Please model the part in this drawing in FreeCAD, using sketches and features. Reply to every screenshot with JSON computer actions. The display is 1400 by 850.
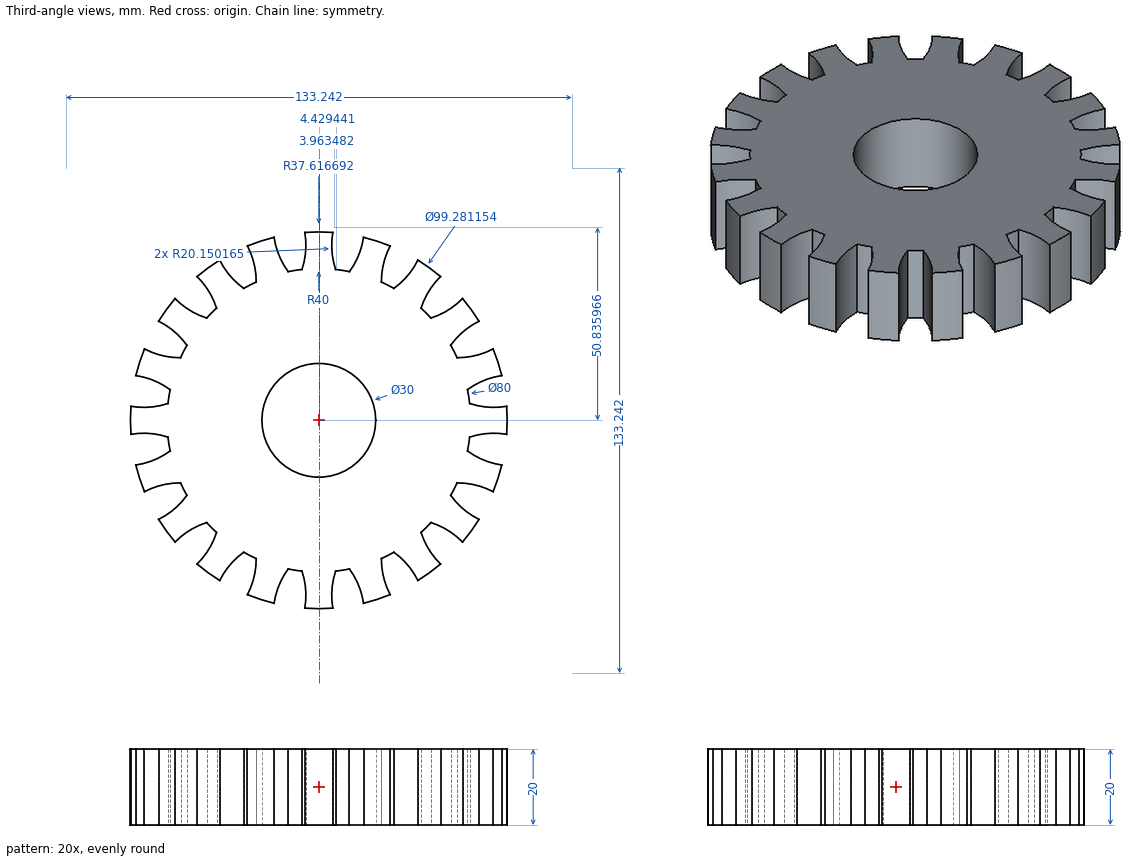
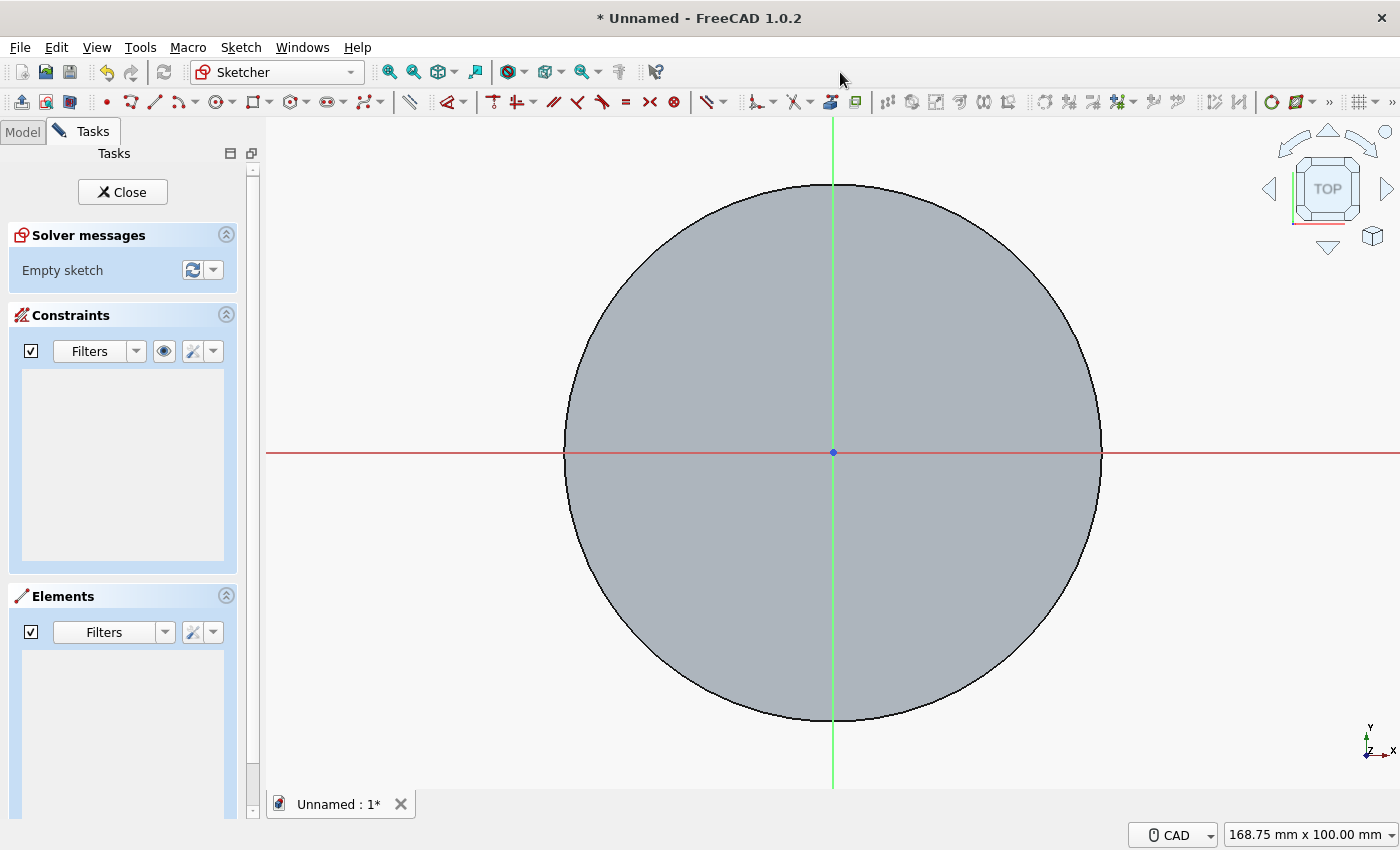
{"action": "scroll", "coordinate": [889, 453], "scroll_direction": "up", "scroll_amount": 4}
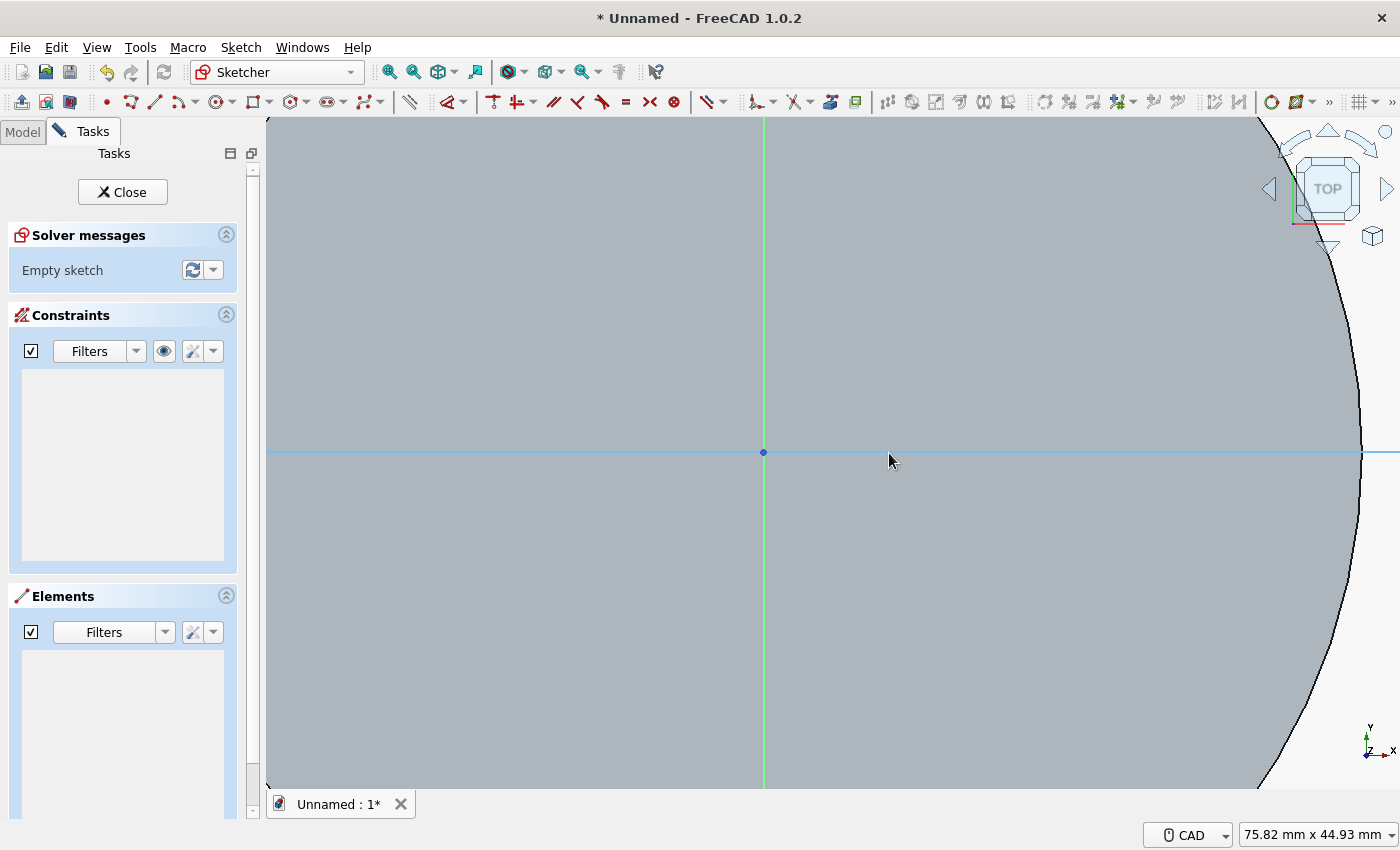
{"action": "left_click", "coordinate": [216, 102]}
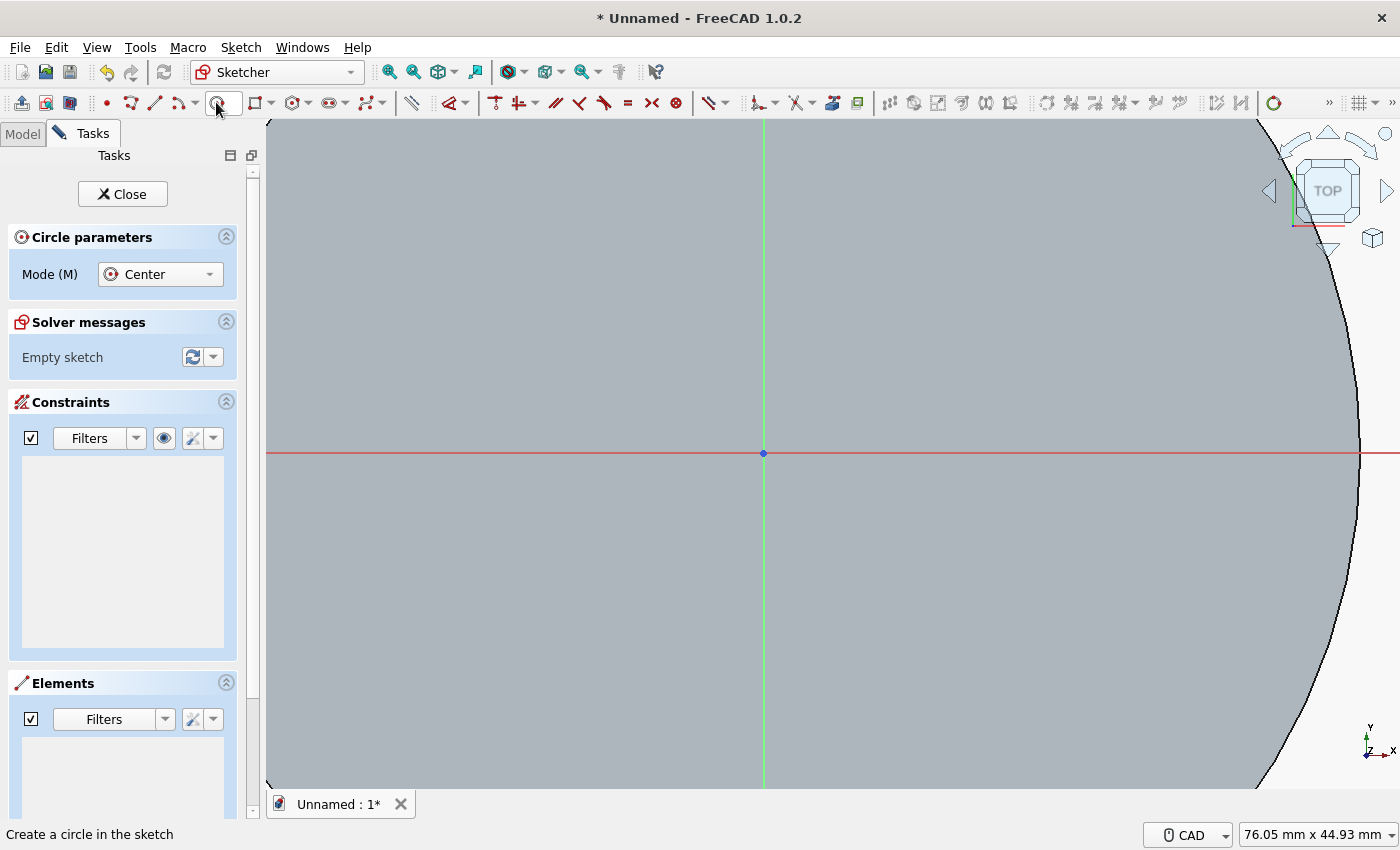
{"action": "left_click", "coordinate": [764, 453]}
{"action": "left_click", "coordinate": [922, 295]}
{"action": "key", "text": "Escape"}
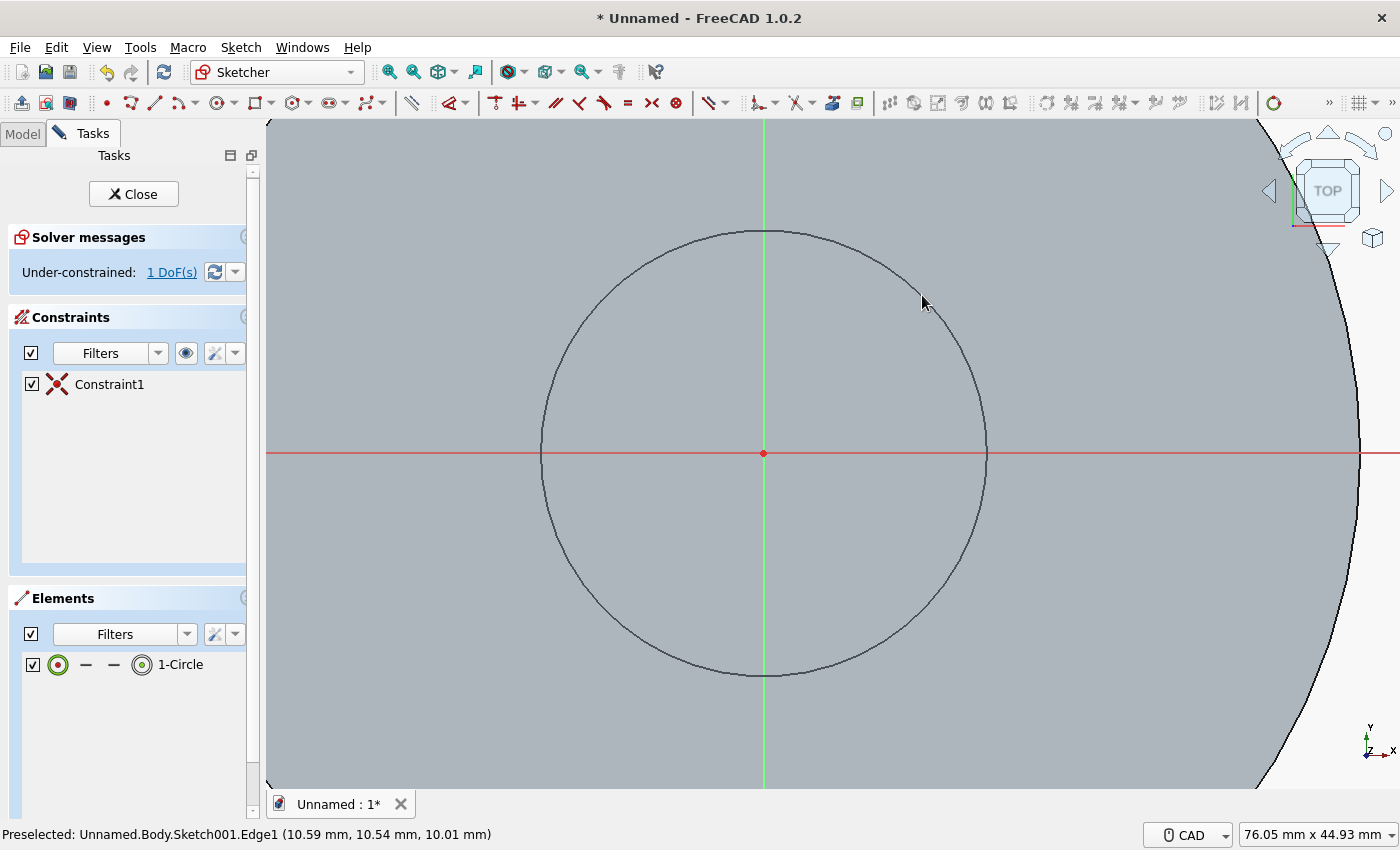
{"action": "left_click", "coordinate": [450, 104]}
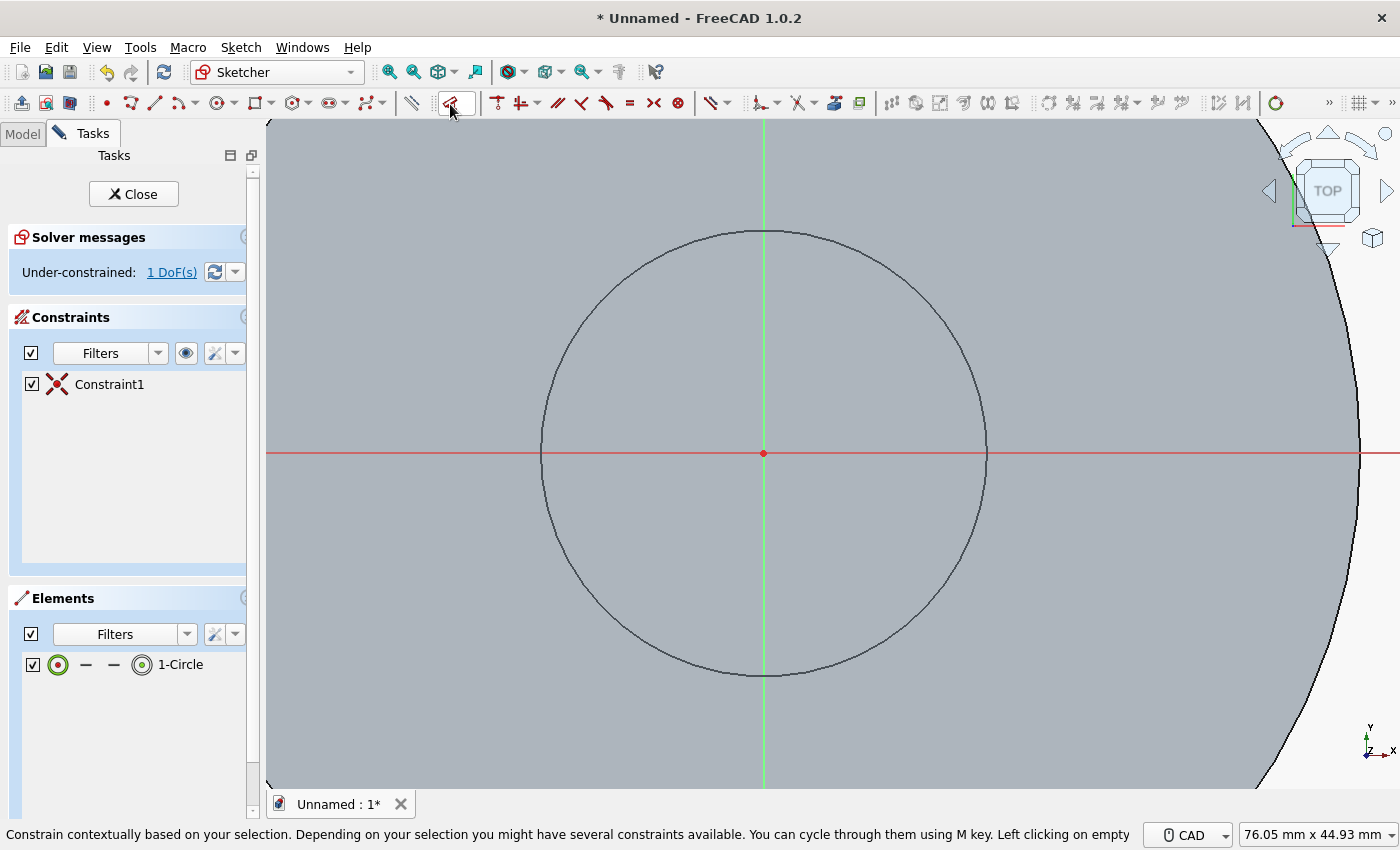
{"action": "left_click", "coordinate": [921, 295]}
{"action": "left_click", "coordinate": [944, 272]}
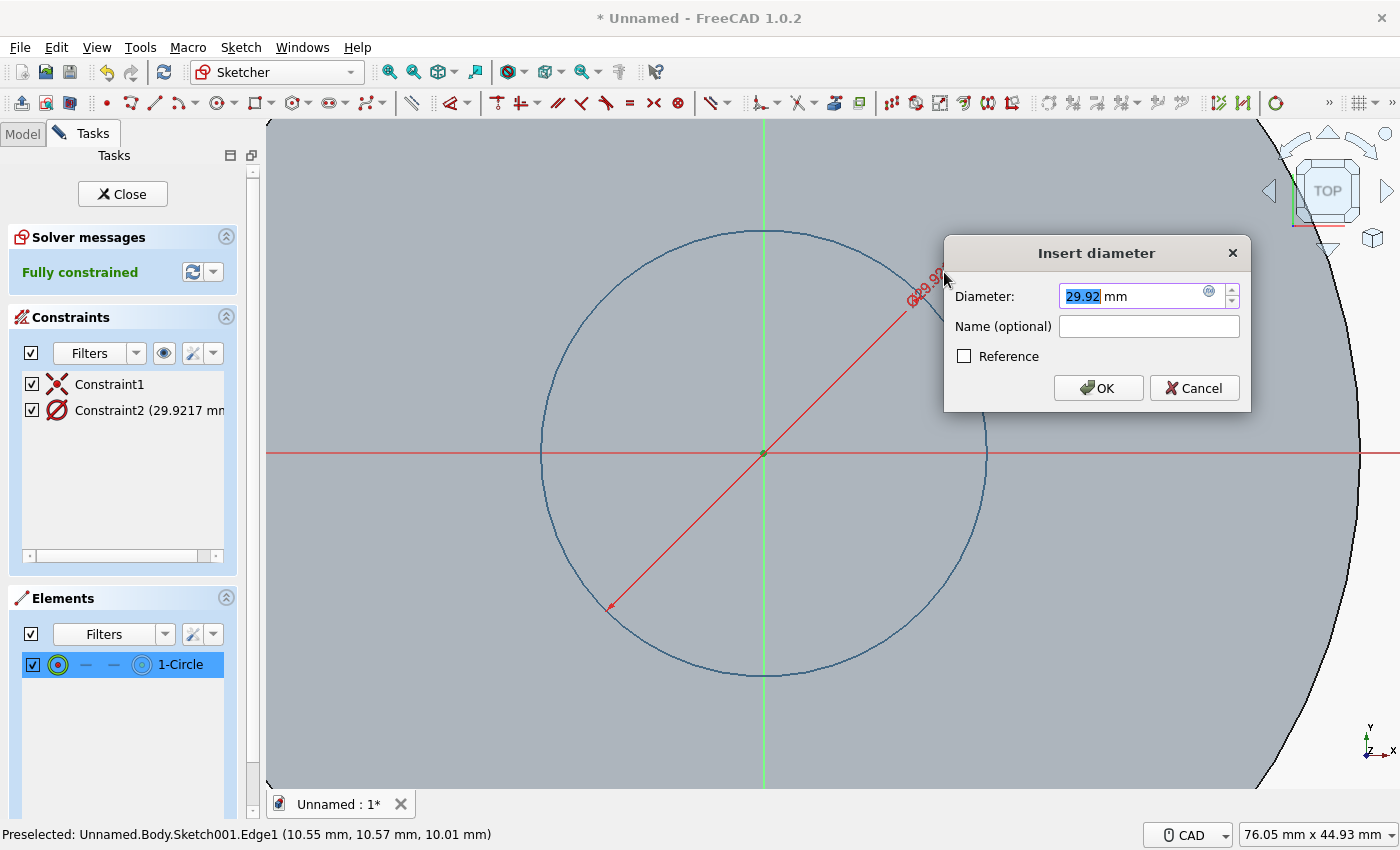
{"action": "type", "text": "30"}
{"action": "key", "text": "Return"}
{"action": "key", "text": "Escape"}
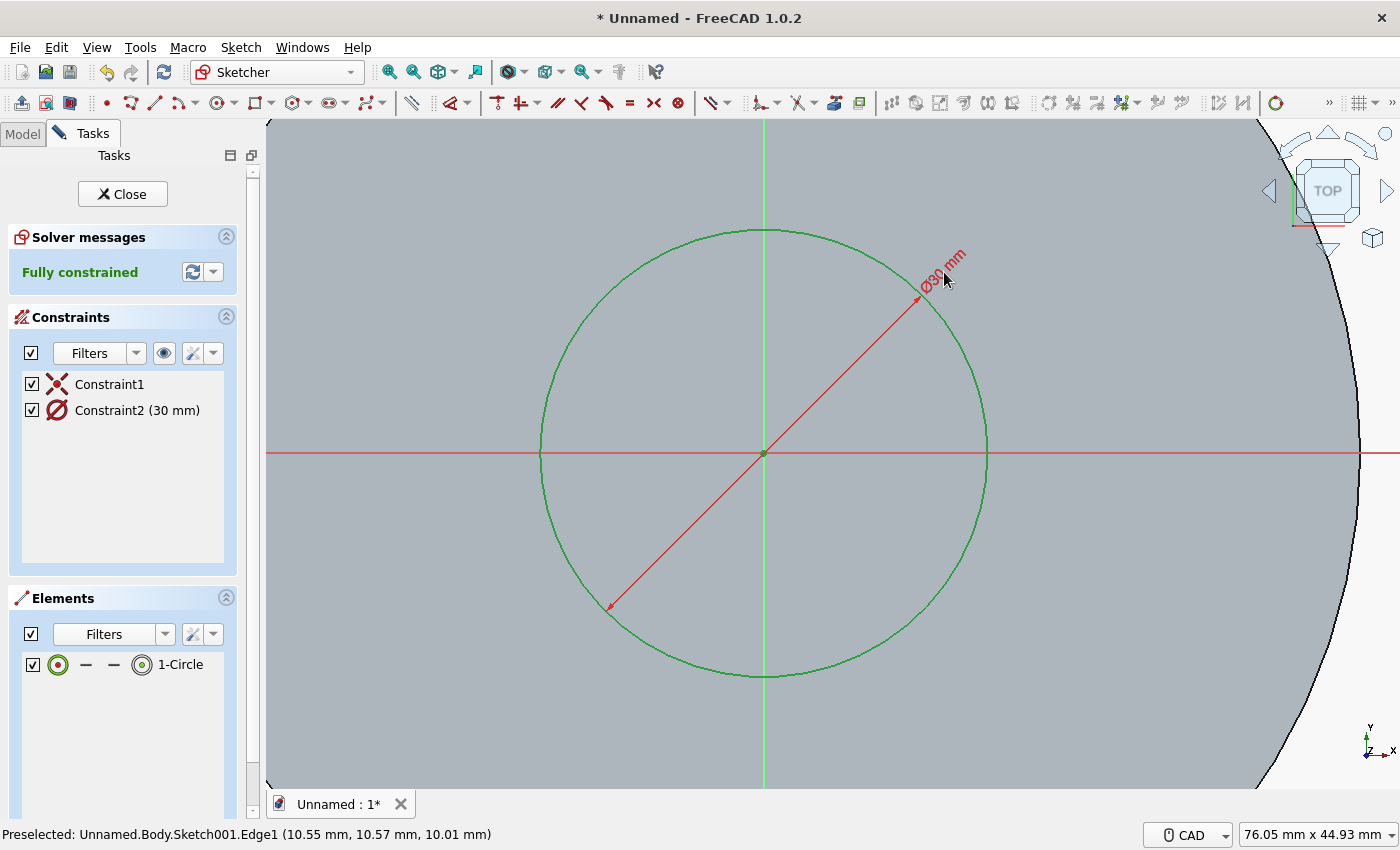
{"action": "left_click", "coordinate": [123, 194]}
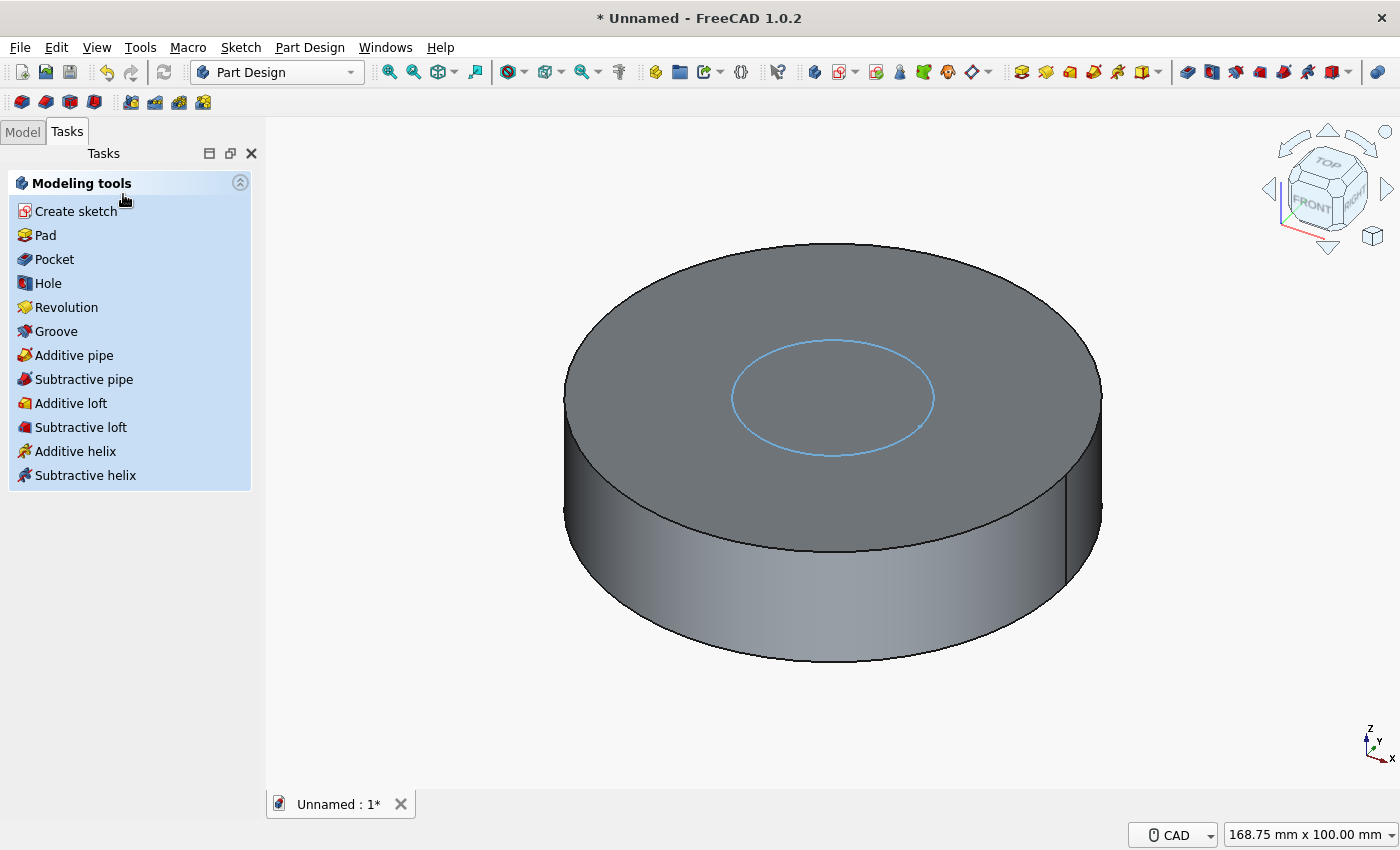
{"action": "left_click", "coordinate": [1188, 72]}